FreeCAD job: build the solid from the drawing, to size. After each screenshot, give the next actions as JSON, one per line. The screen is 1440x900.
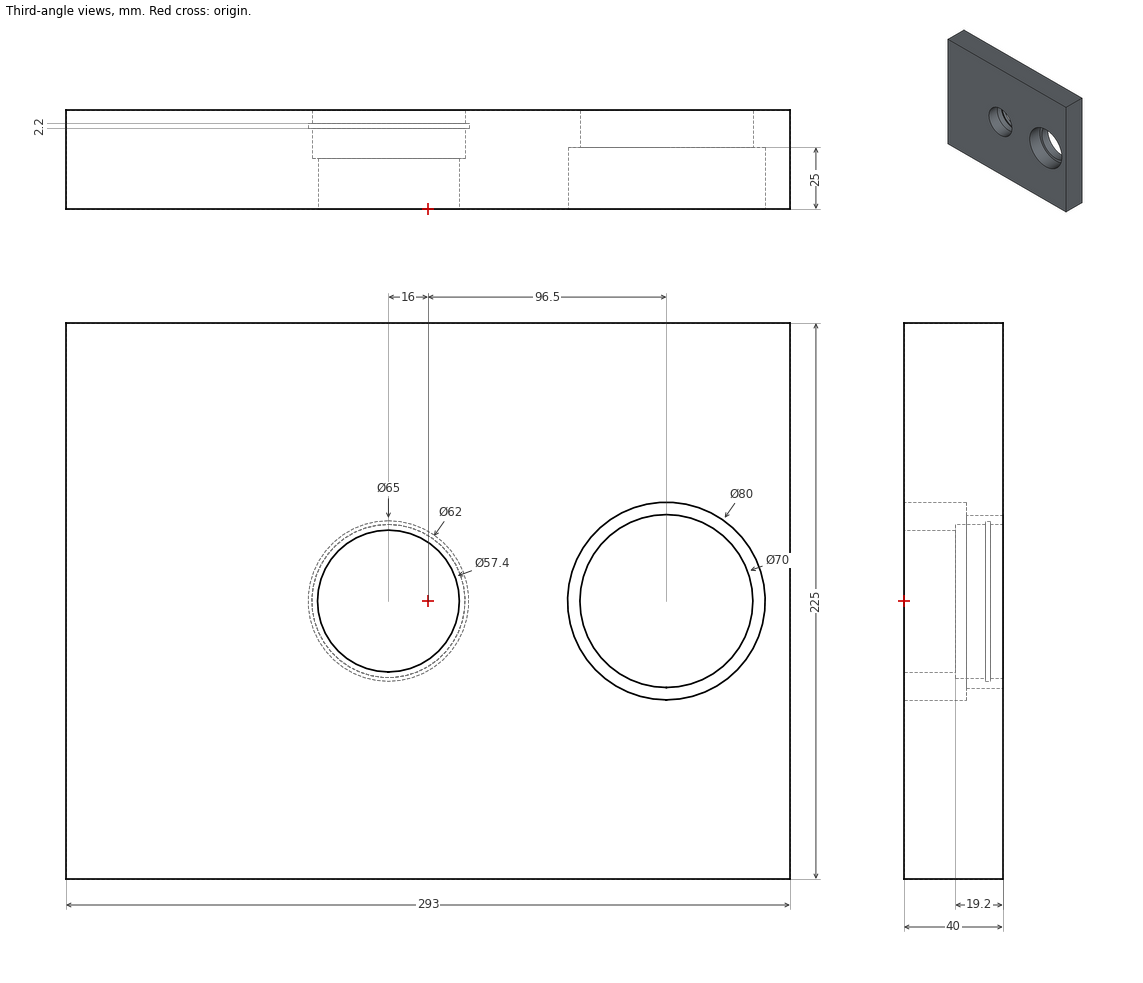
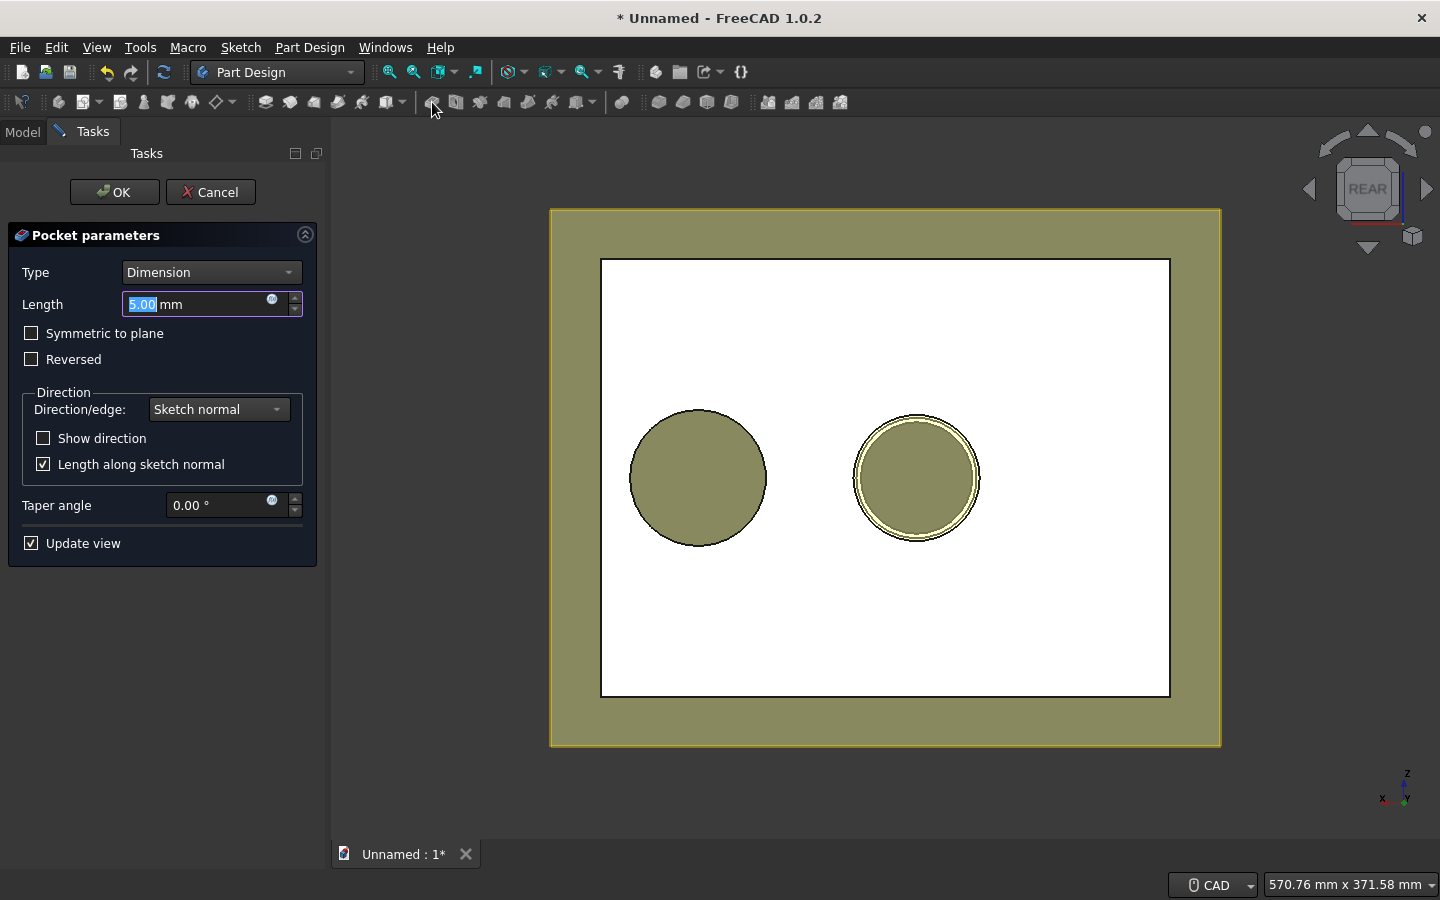
{"action": "type", "text": "2.2"}
{"action": "key", "text": "Tab"}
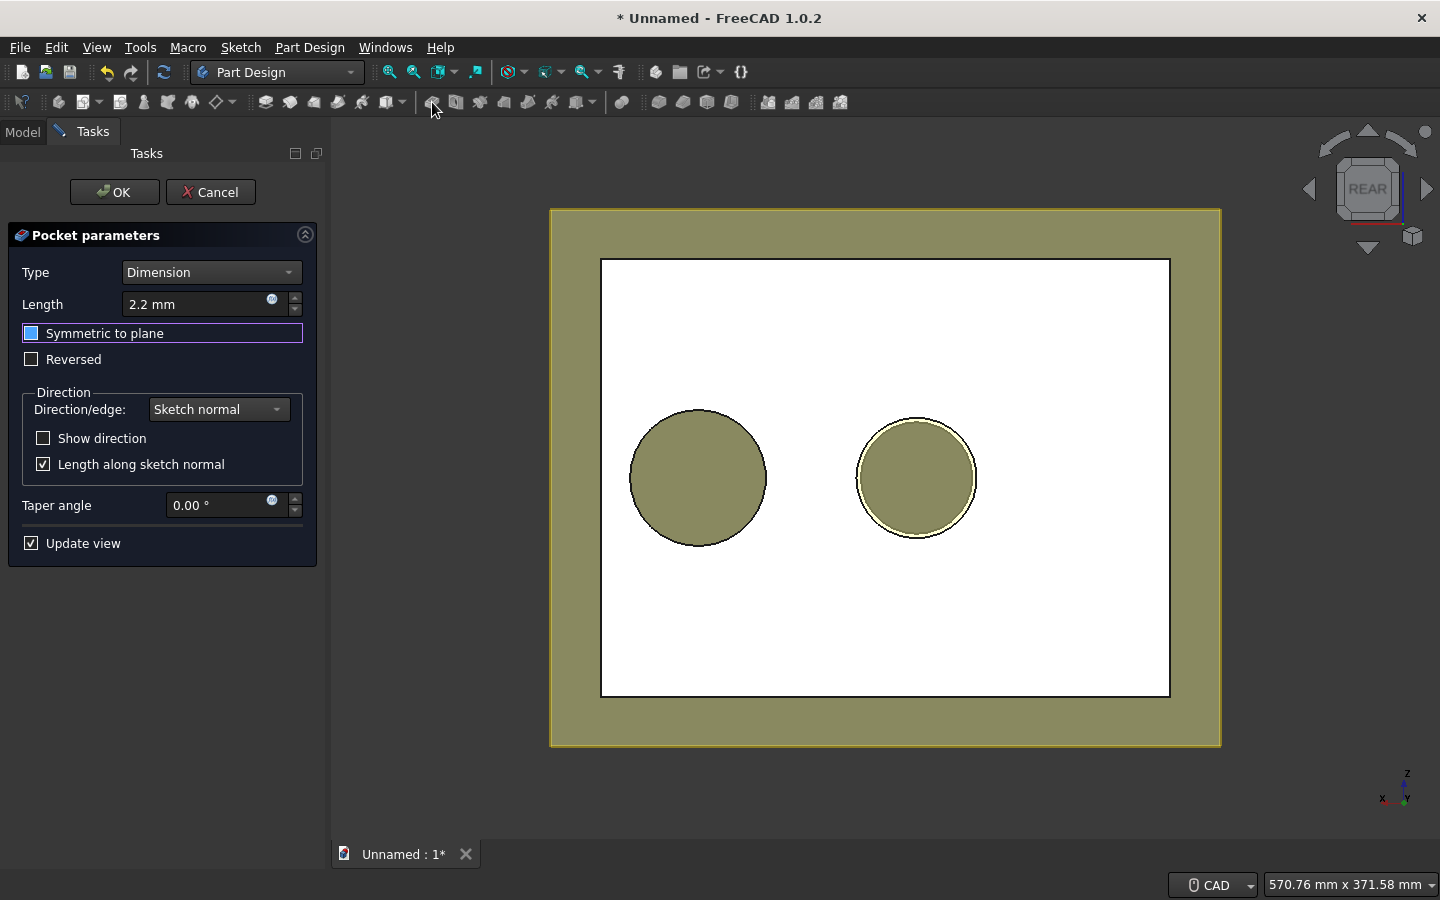
{"action": "left_click", "coordinate": [30, 359]}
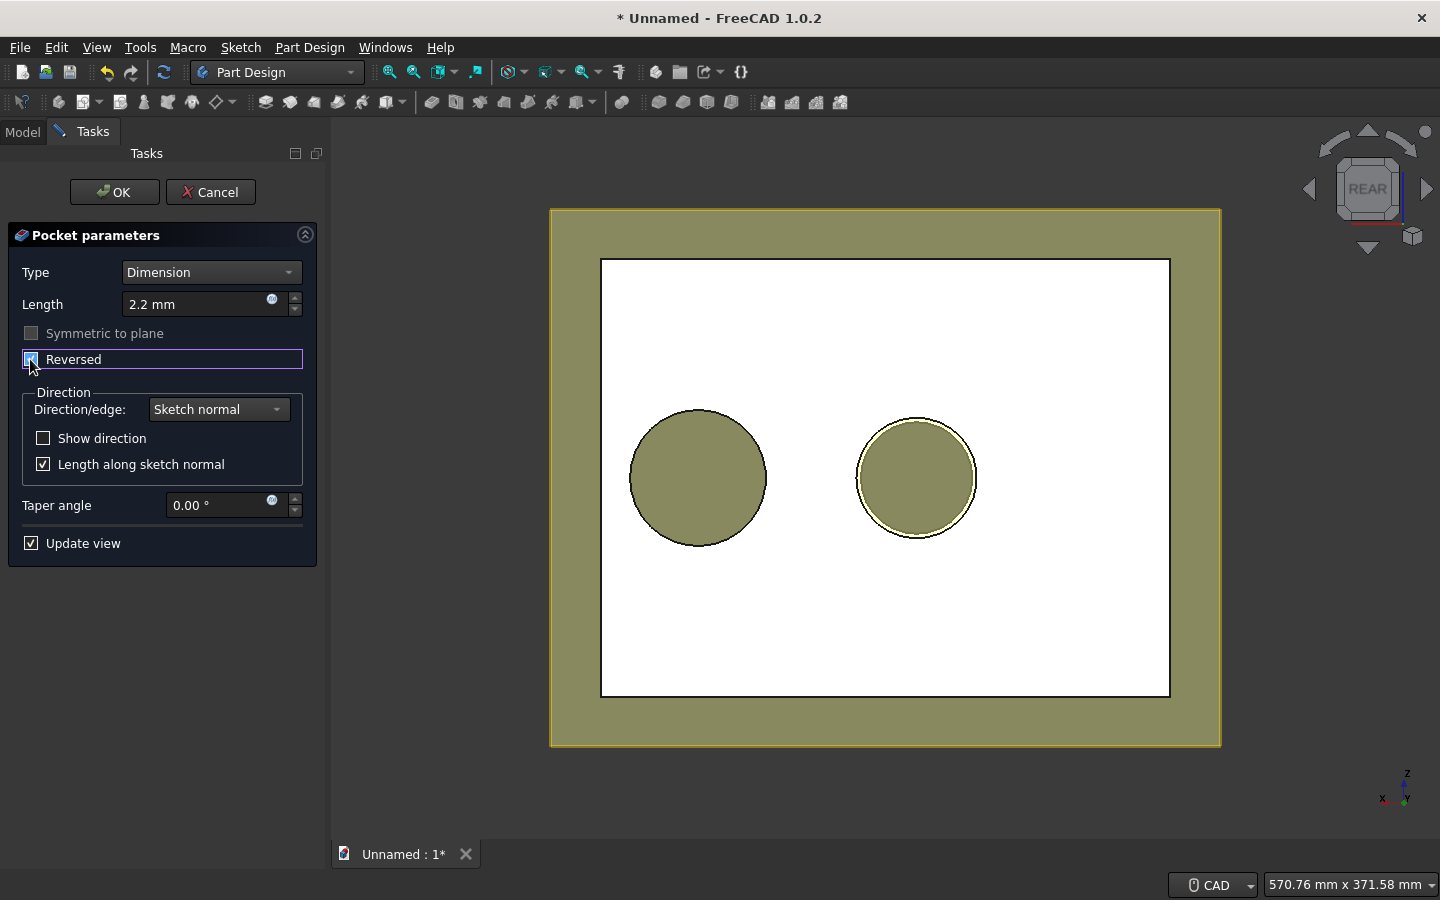
{"action": "left_click", "coordinate": [115, 192]}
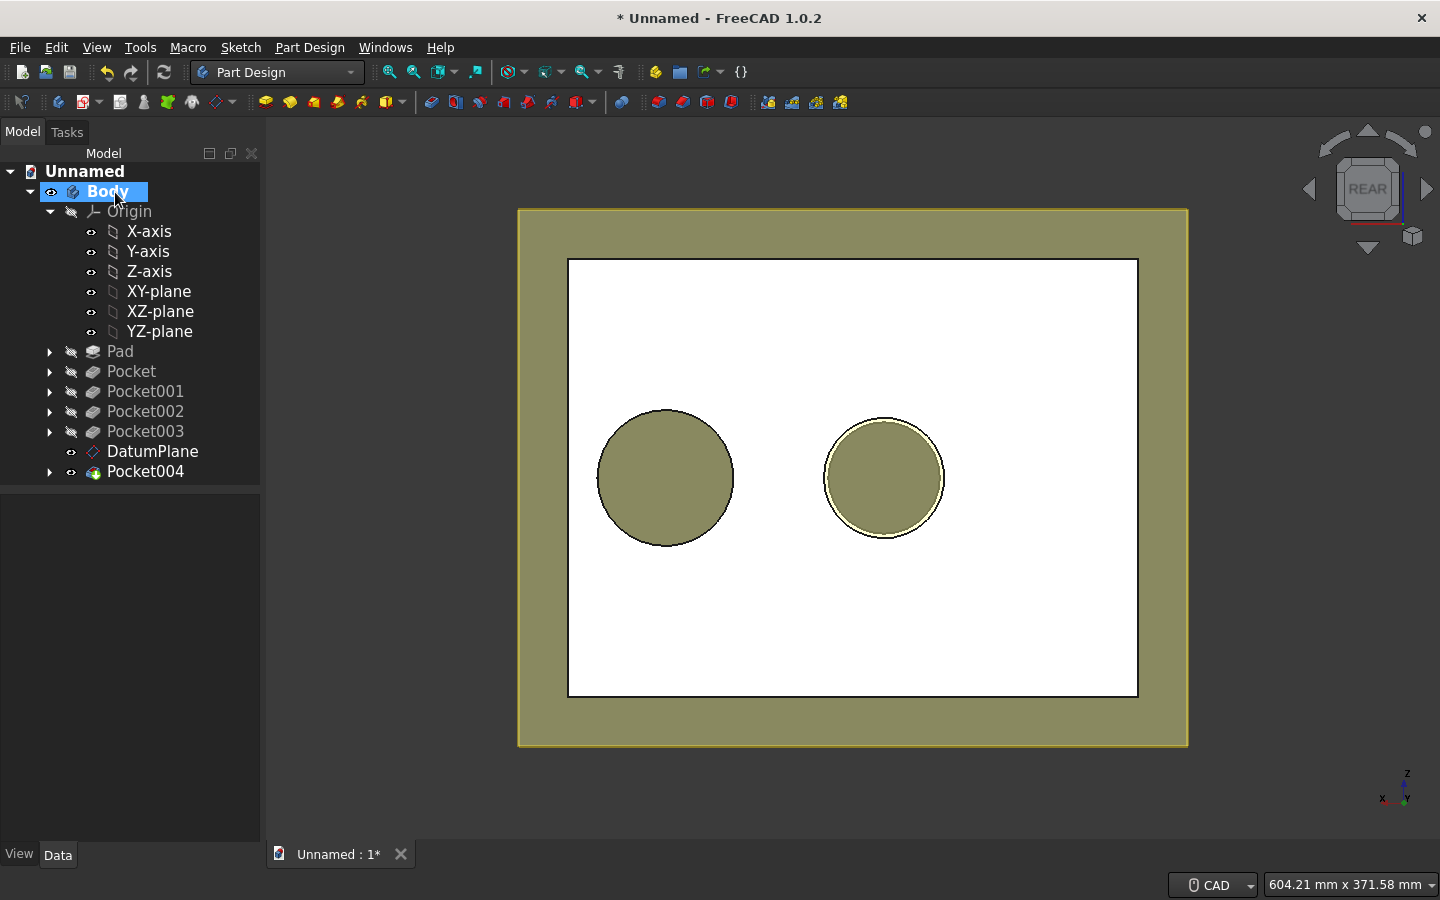
{"action": "left_click", "coordinate": [116, 452]}
{"action": "key", "text": "space"}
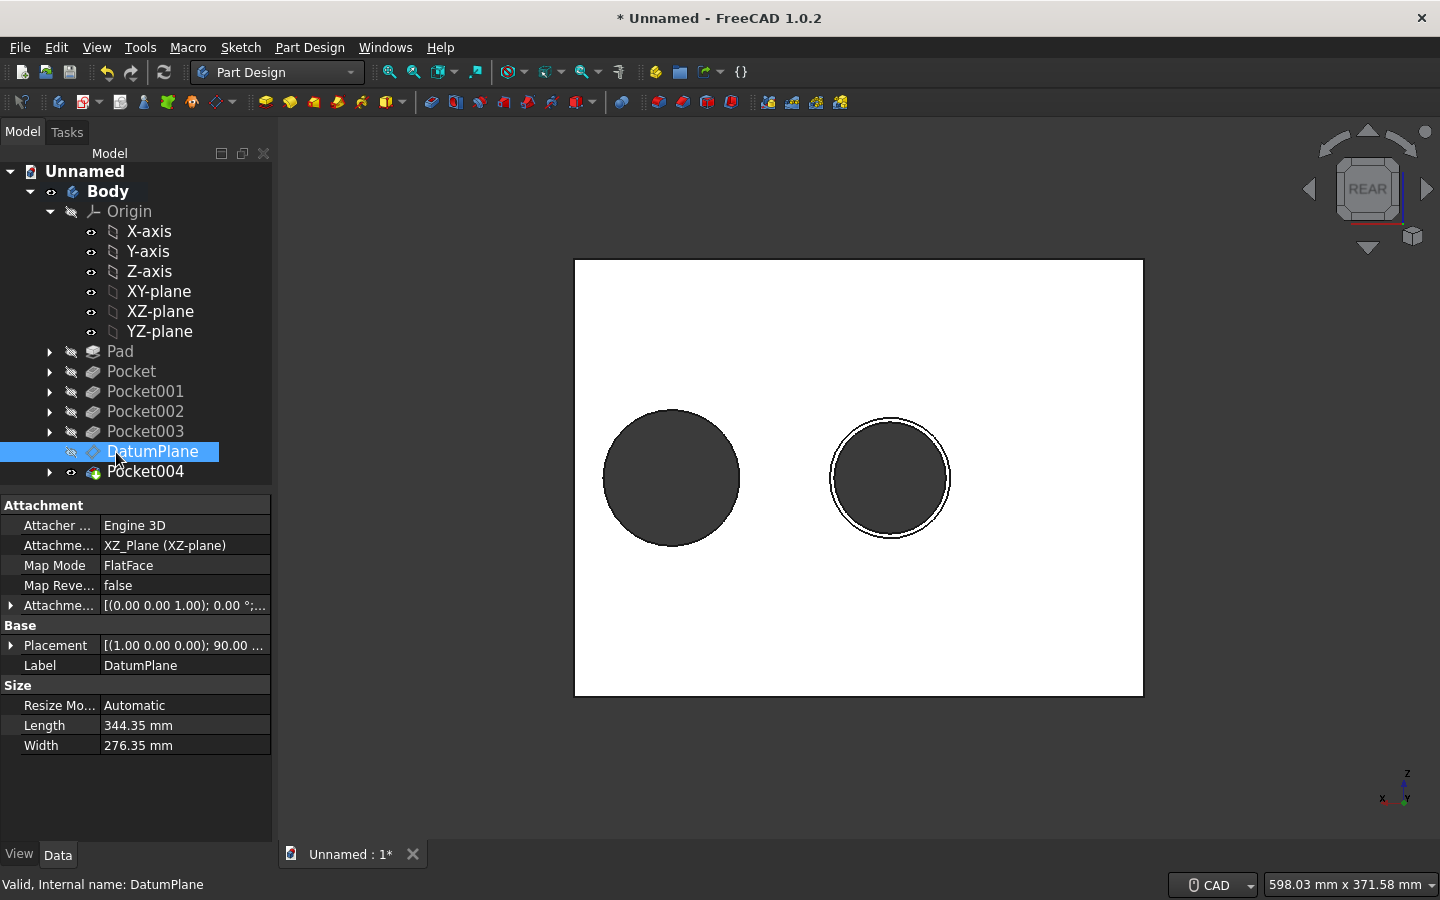
{"action": "key", "text": "0"}